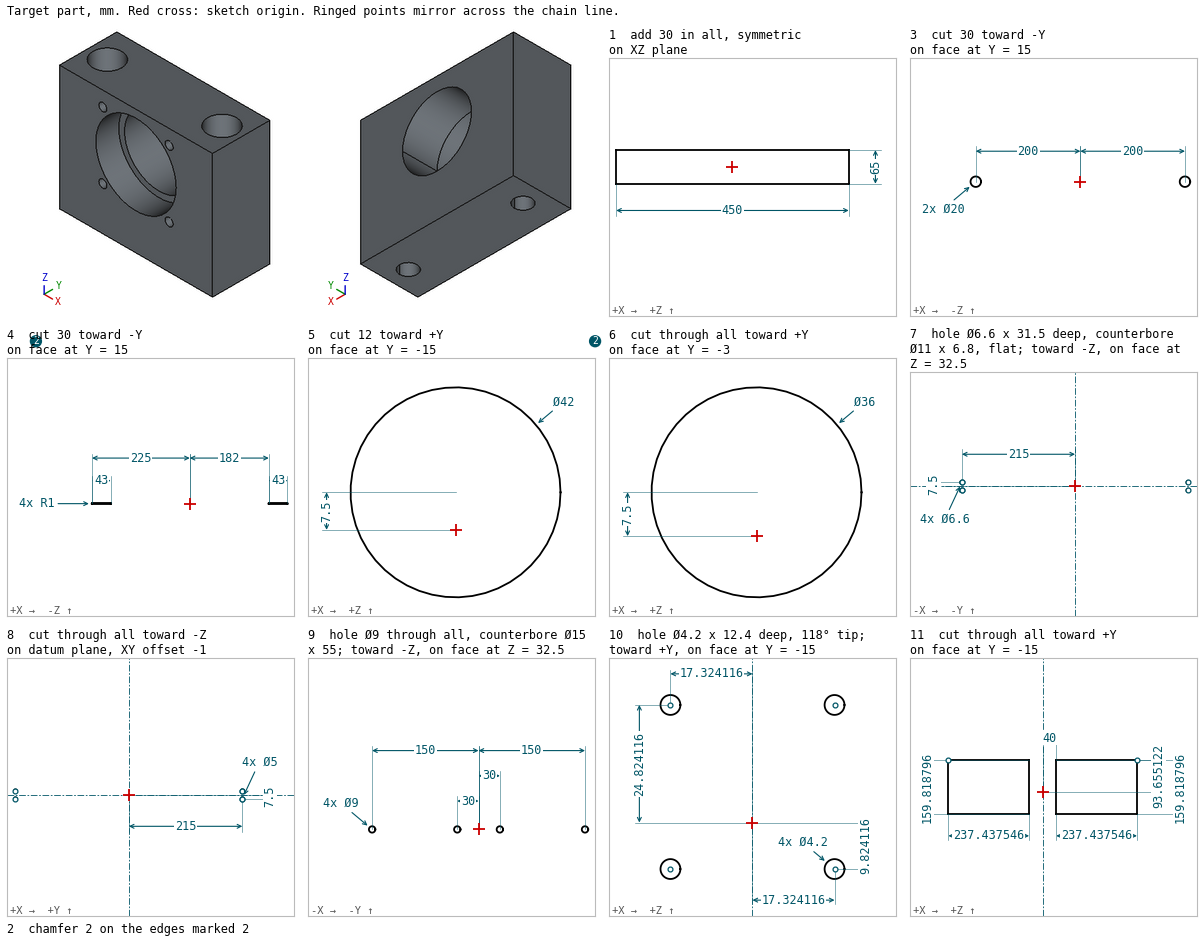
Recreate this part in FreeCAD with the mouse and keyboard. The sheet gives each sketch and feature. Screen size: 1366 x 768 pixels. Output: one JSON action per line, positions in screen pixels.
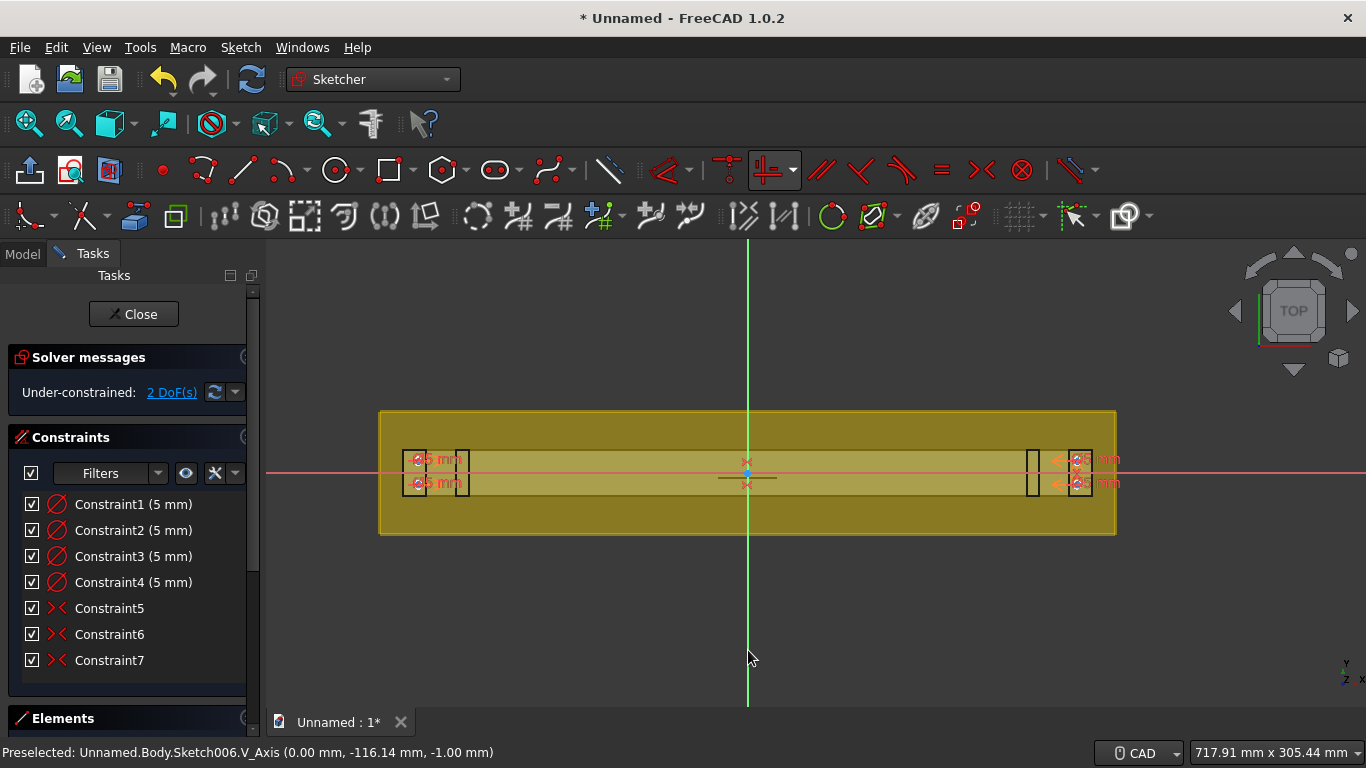
{"action": "key", "text": "d"}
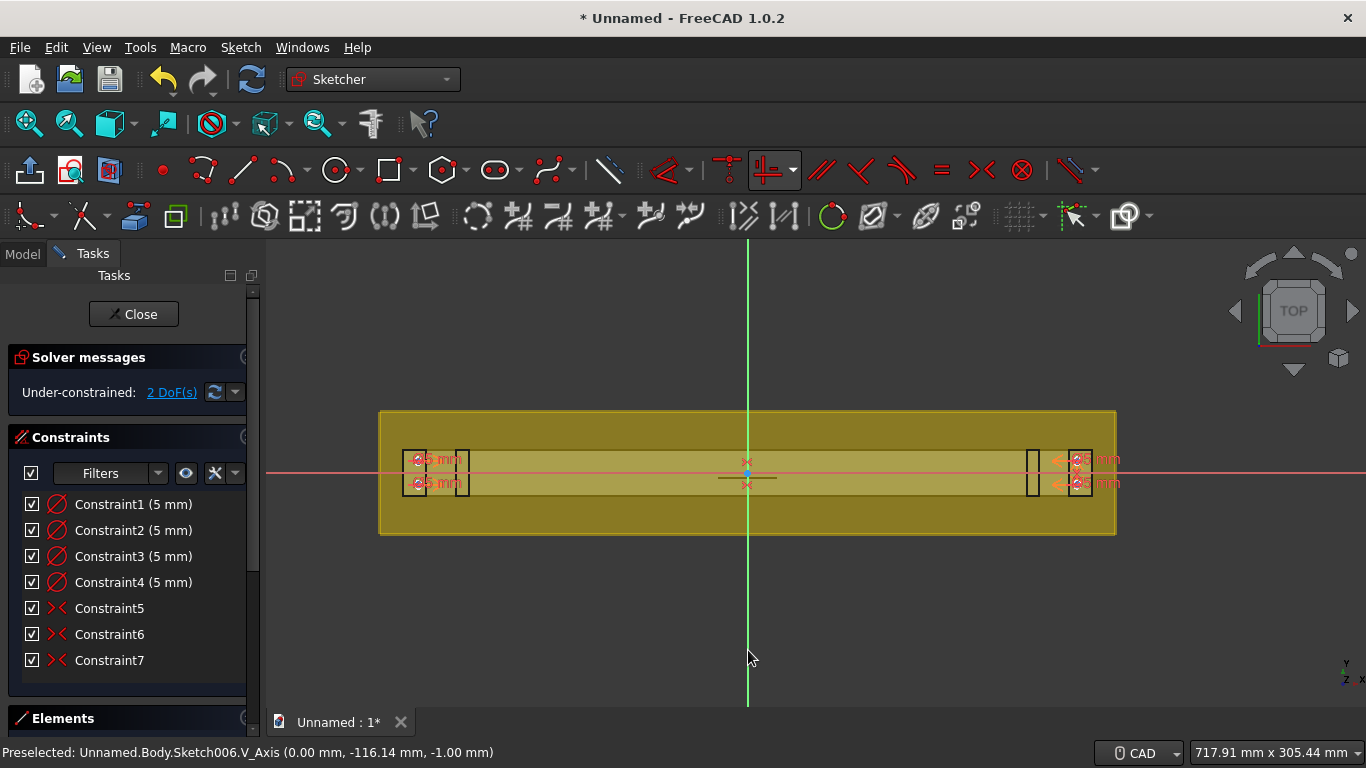
{"action": "left_click", "coordinate": [1077, 485]}
{"action": "left_click", "coordinate": [912, 519]}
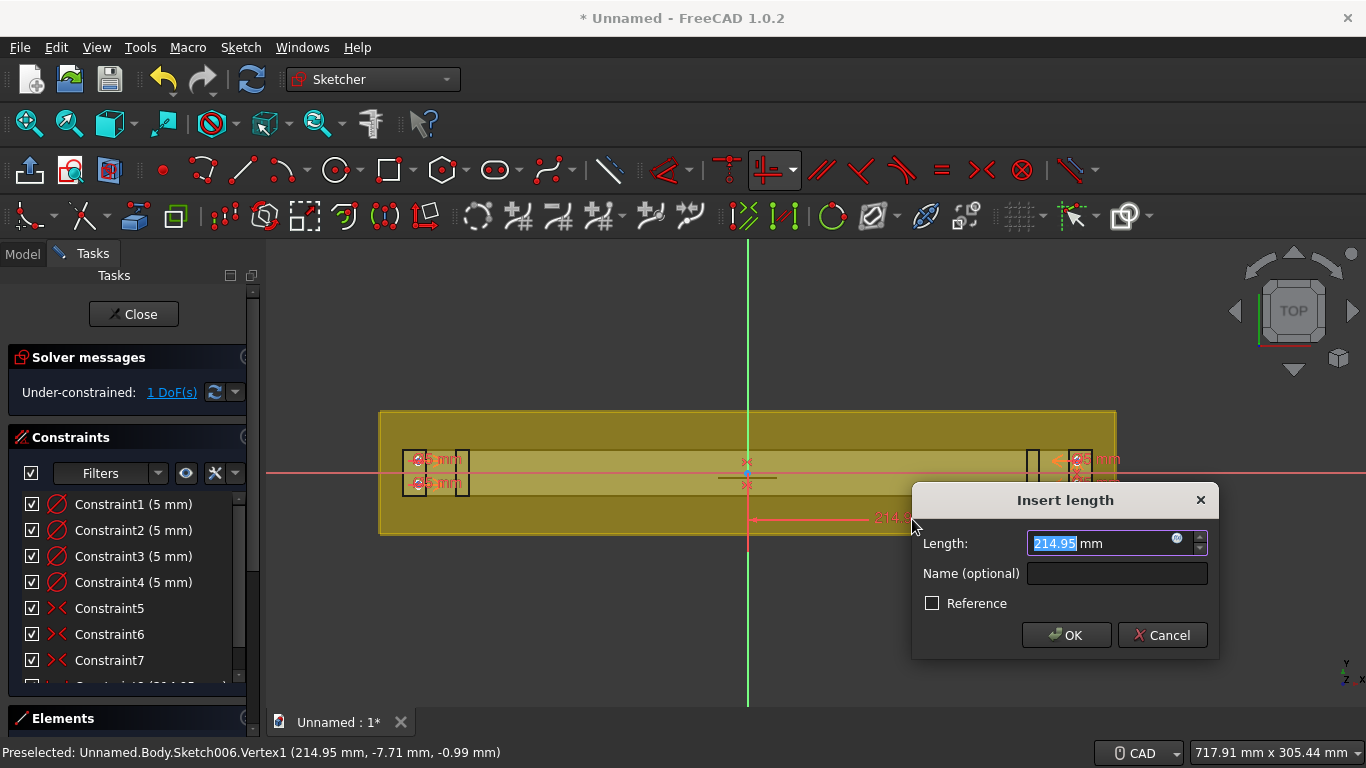
{"action": "type", "text": "215"}
{"action": "key", "text": "Return"}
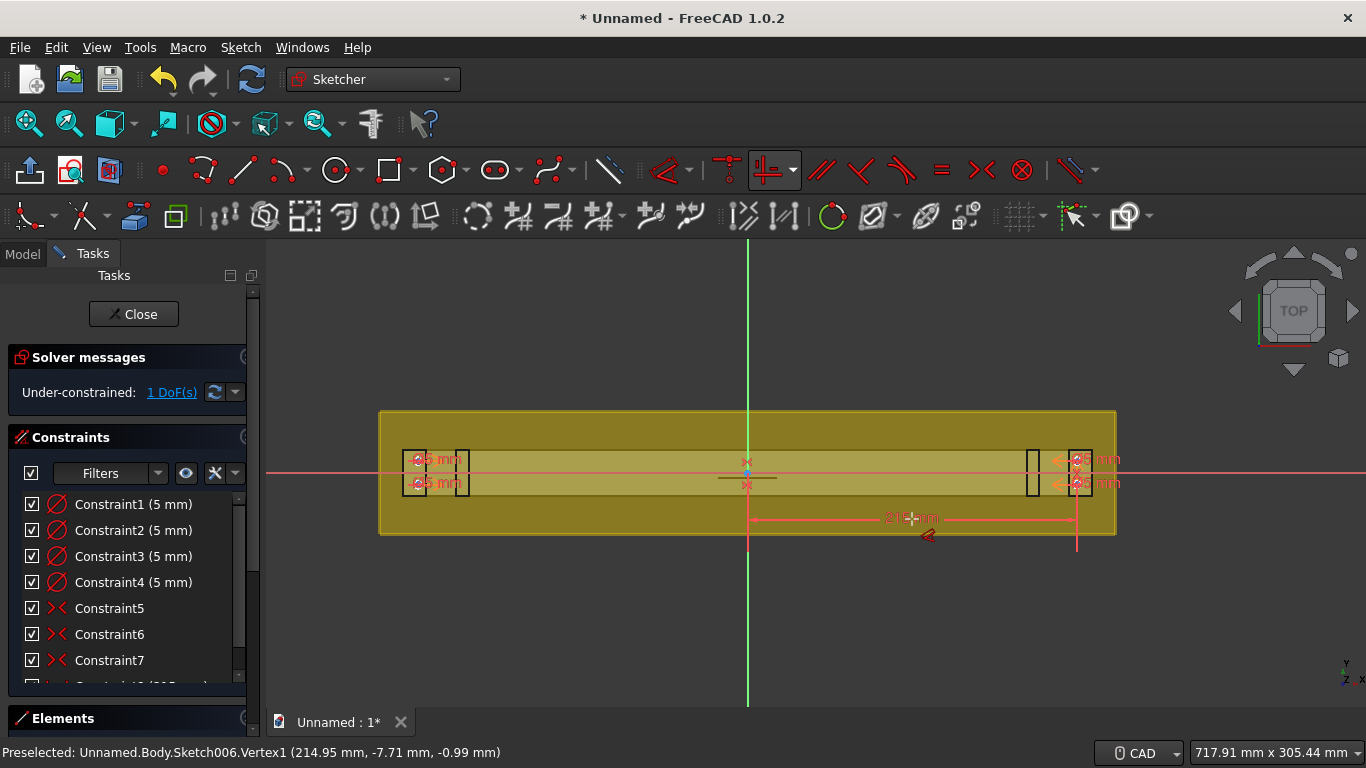
{"action": "scroll", "coordinate": [1077, 485], "scroll_direction": "up", "scroll_amount": 7}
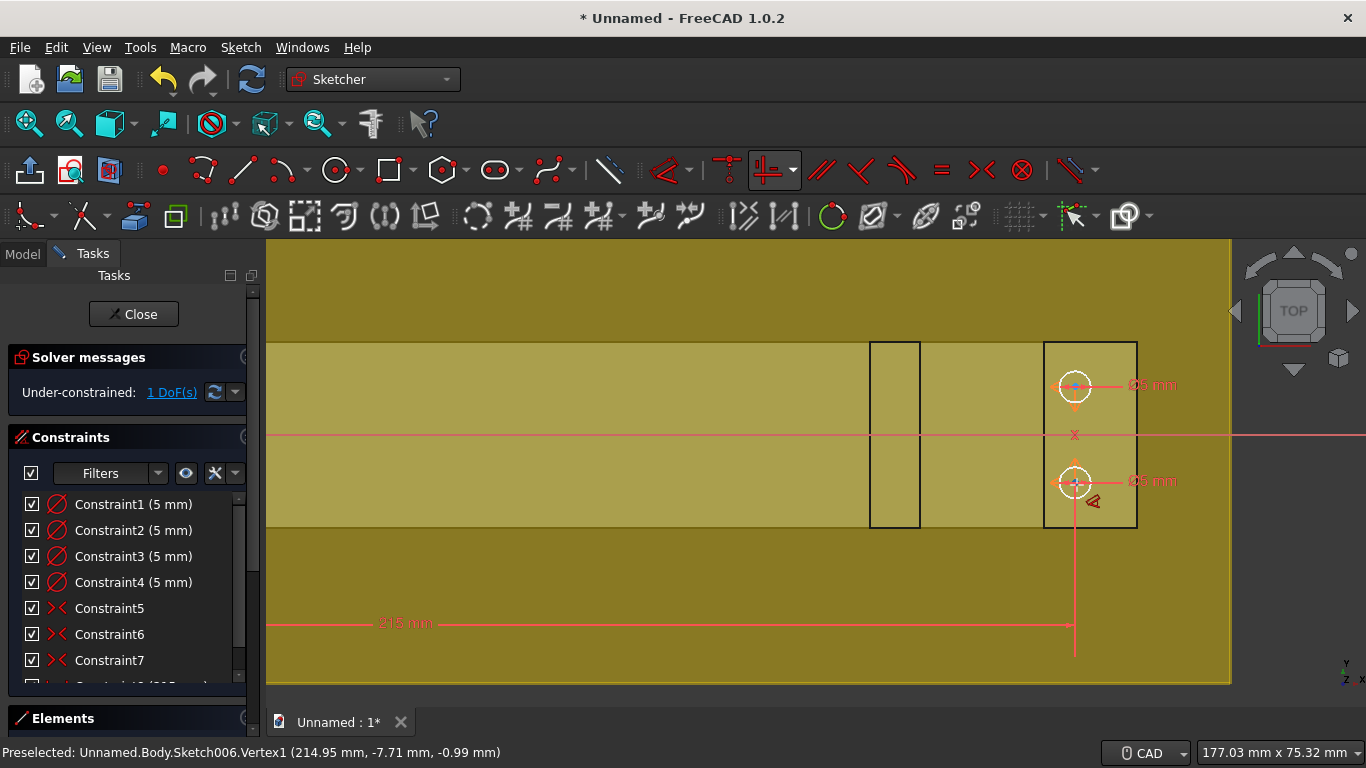
{"action": "left_click", "coordinate": [1075, 483]}
{"action": "left_click", "coordinate": [1109, 459]}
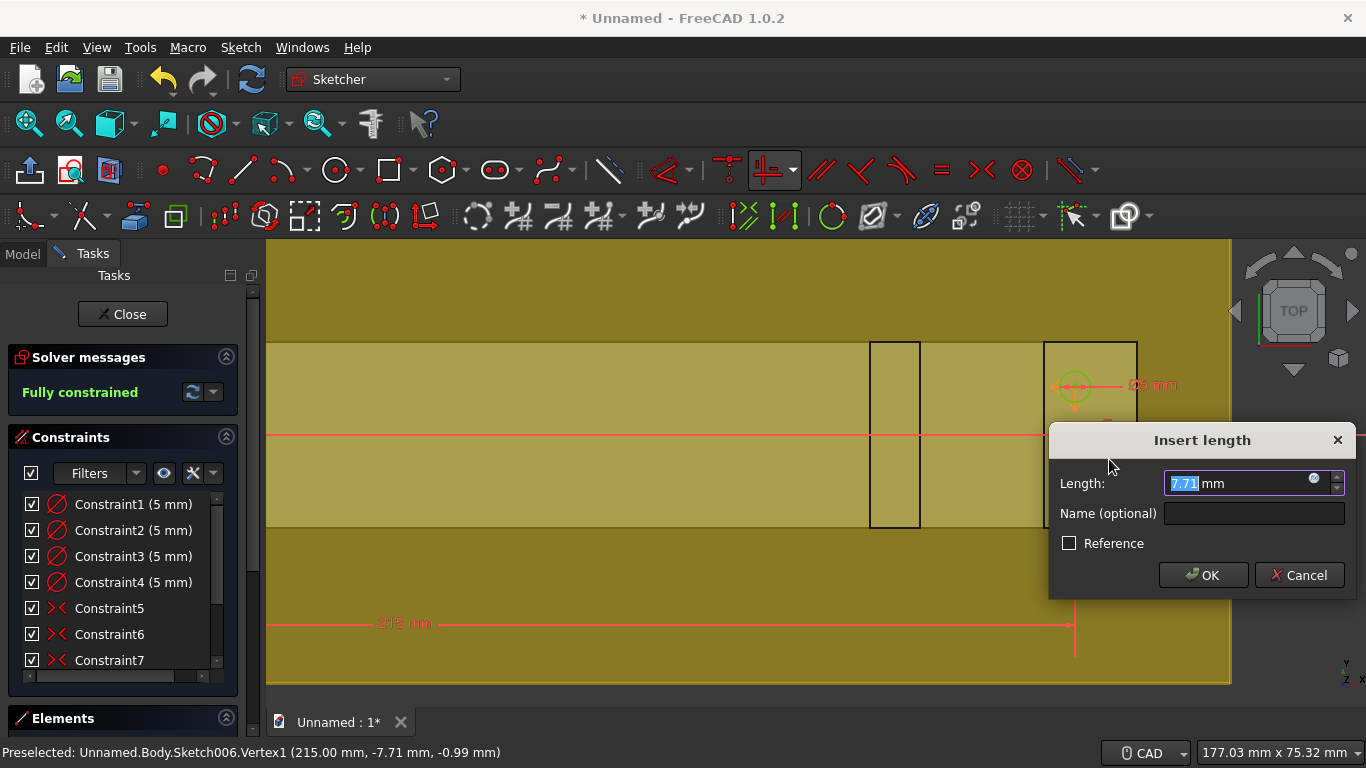
{"action": "type", "text": "7.5"}
{"action": "key", "text": "Return"}
{"action": "key", "text": "Escape"}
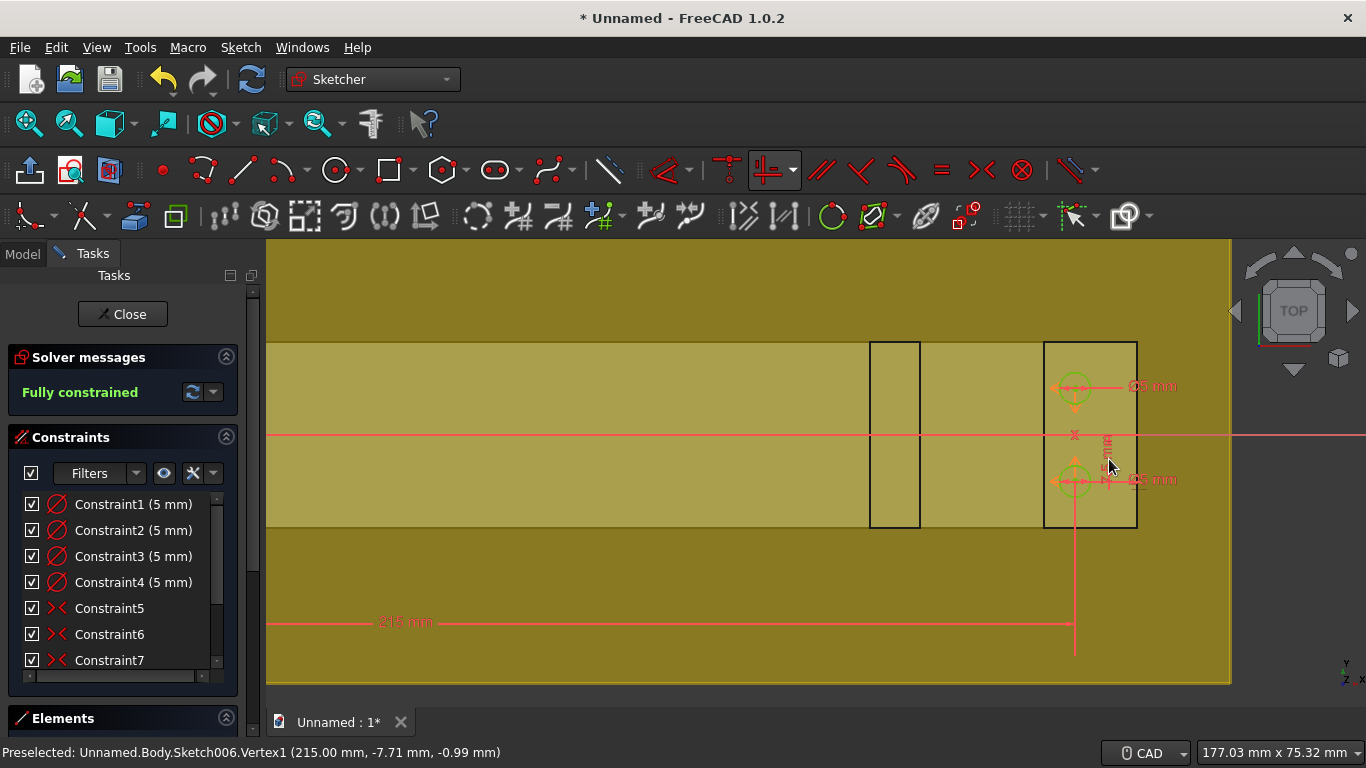
{"action": "left_click", "coordinate": [123, 314]}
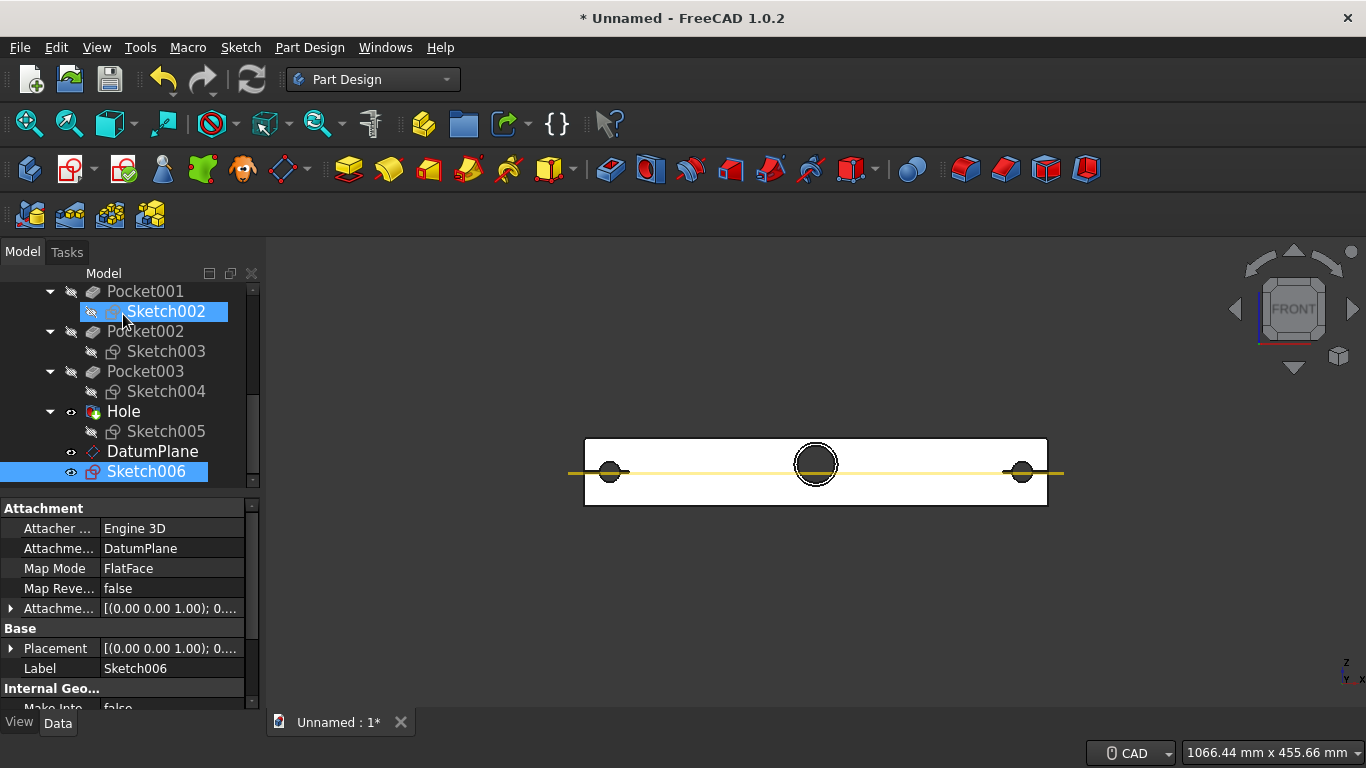
{"action": "left_click", "coordinate": [612, 170]}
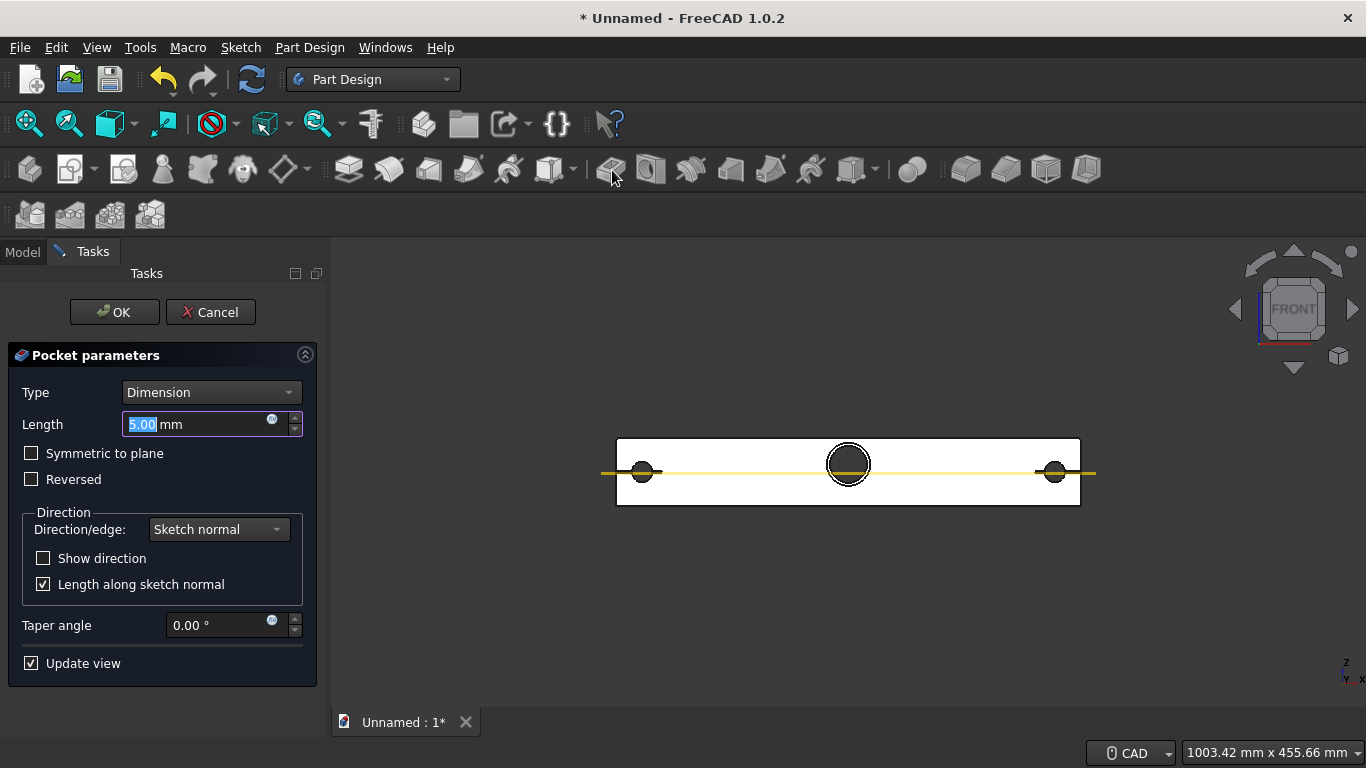
{"action": "left_click", "coordinate": [212, 392]}